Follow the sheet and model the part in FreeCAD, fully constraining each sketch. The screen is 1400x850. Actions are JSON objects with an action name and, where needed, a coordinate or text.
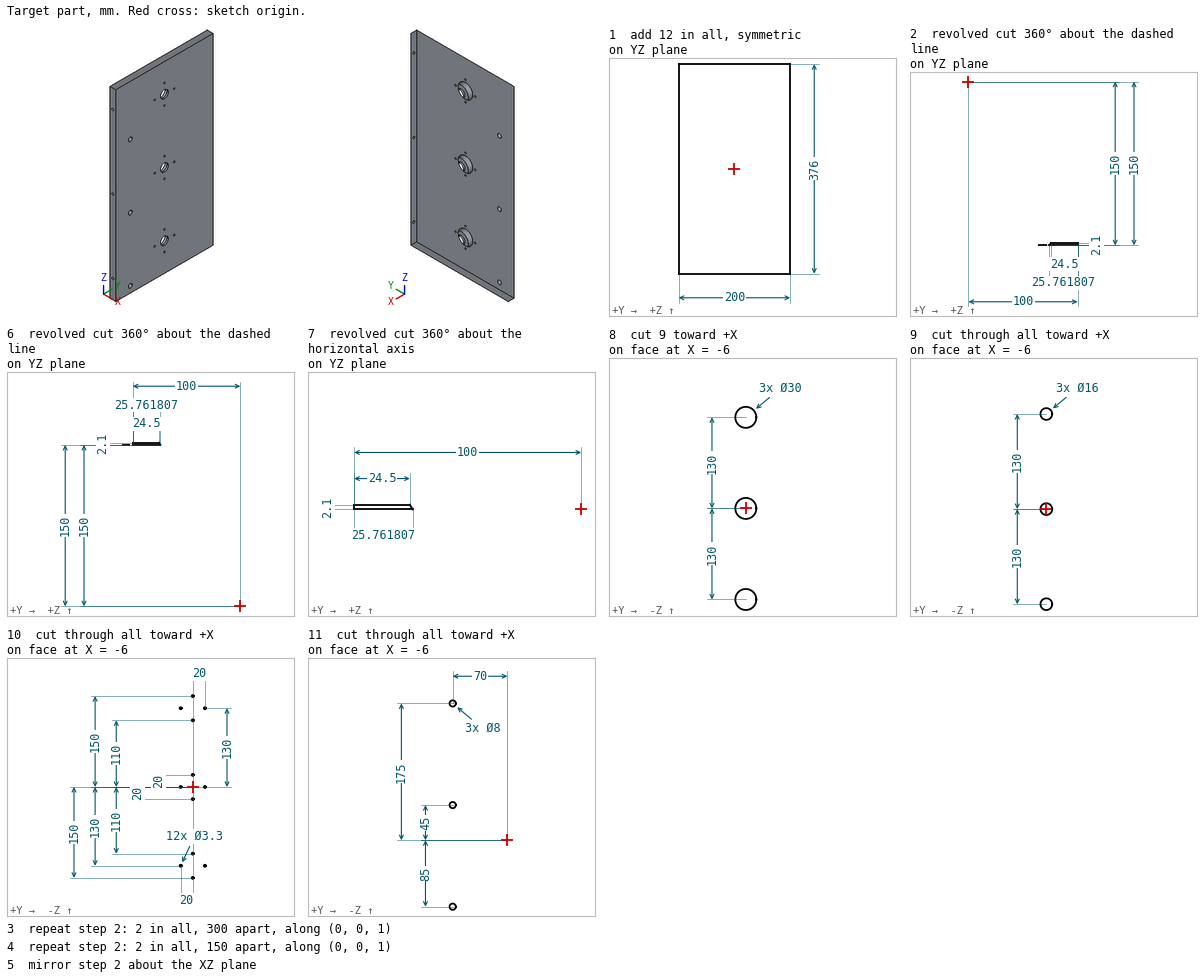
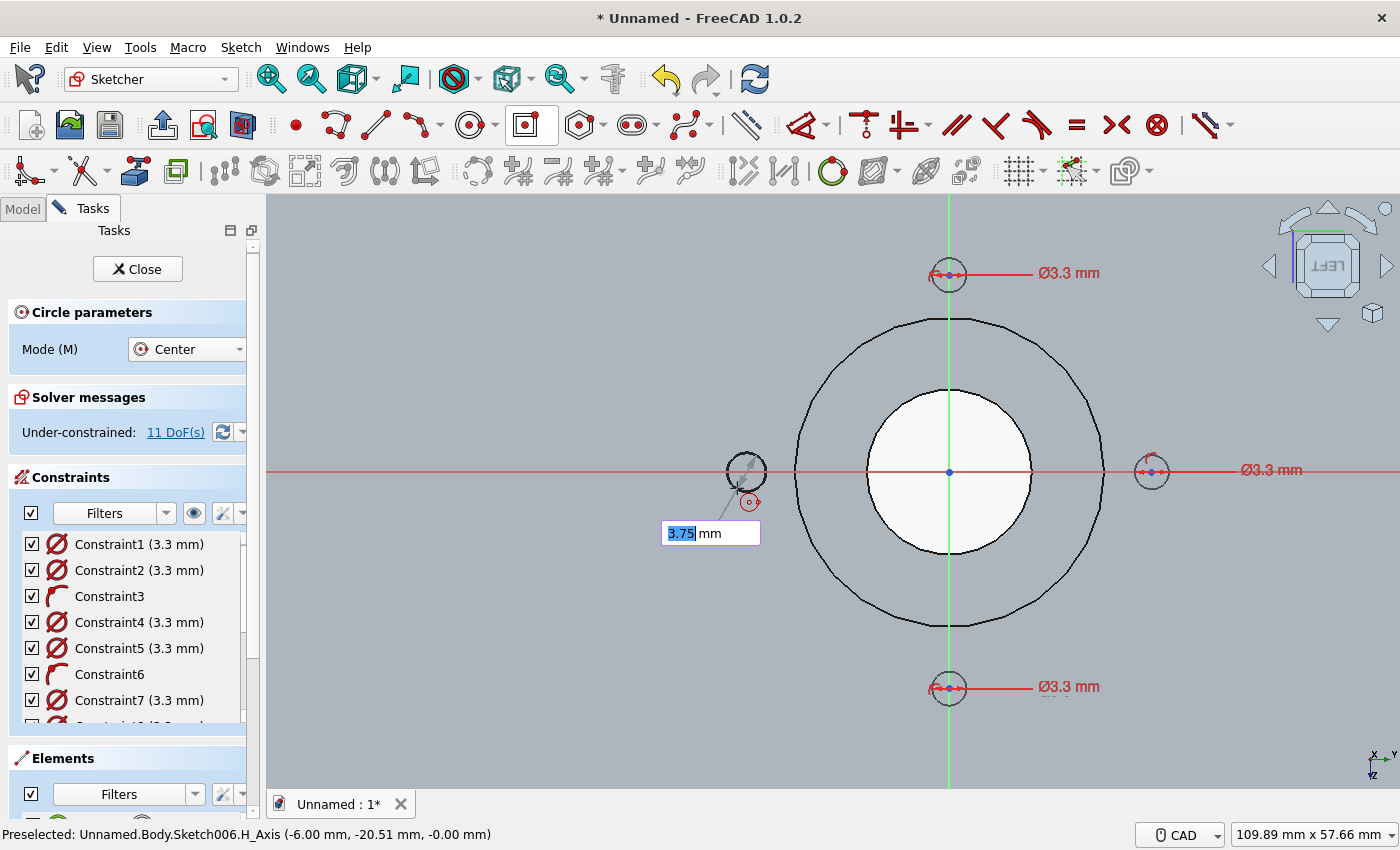
{"action": "type", "text": "3.3"}
{"action": "key", "text": "Return"}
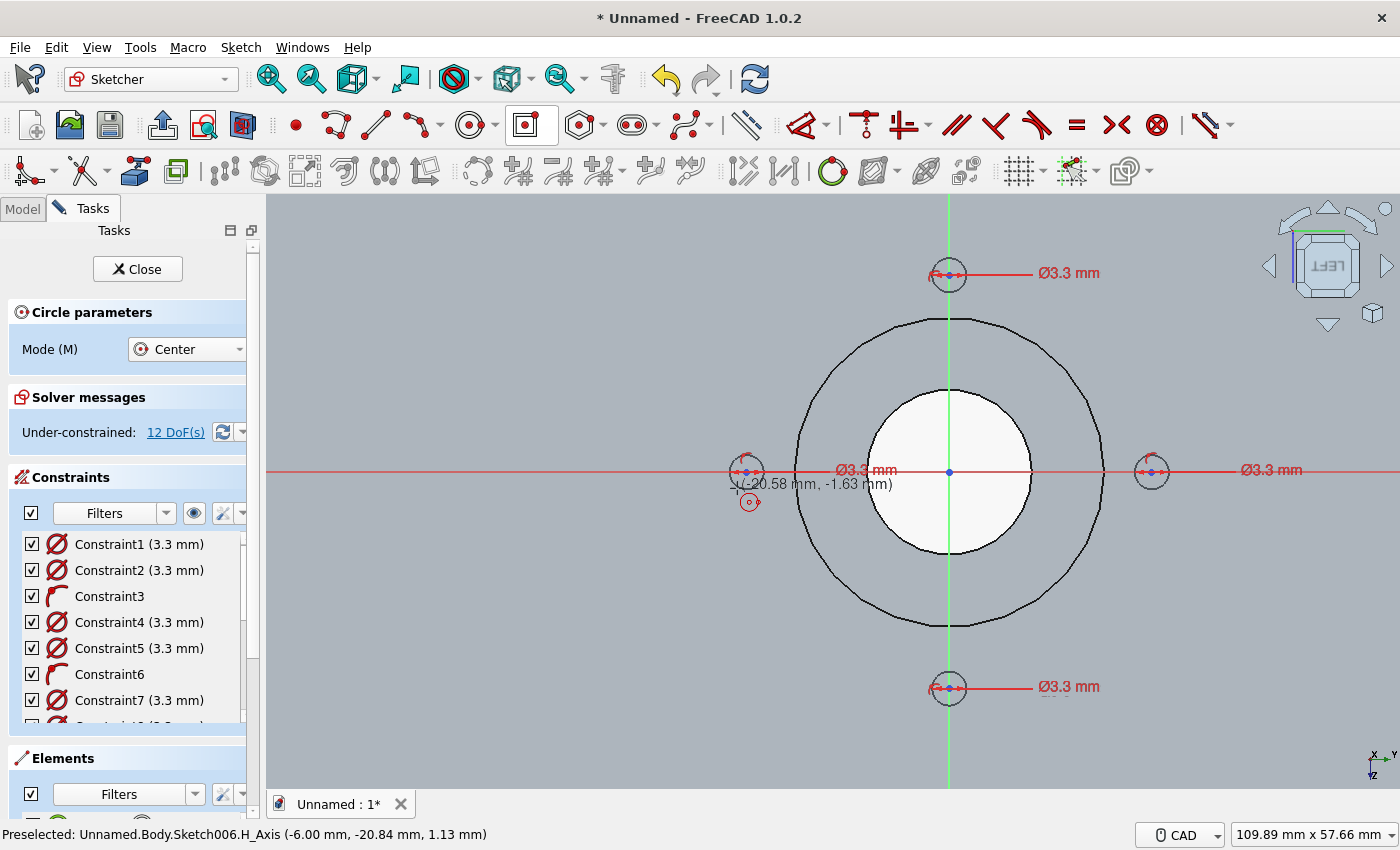
{"action": "scroll", "coordinate": [741, 494], "scroll_direction": "down", "scroll_amount": 11}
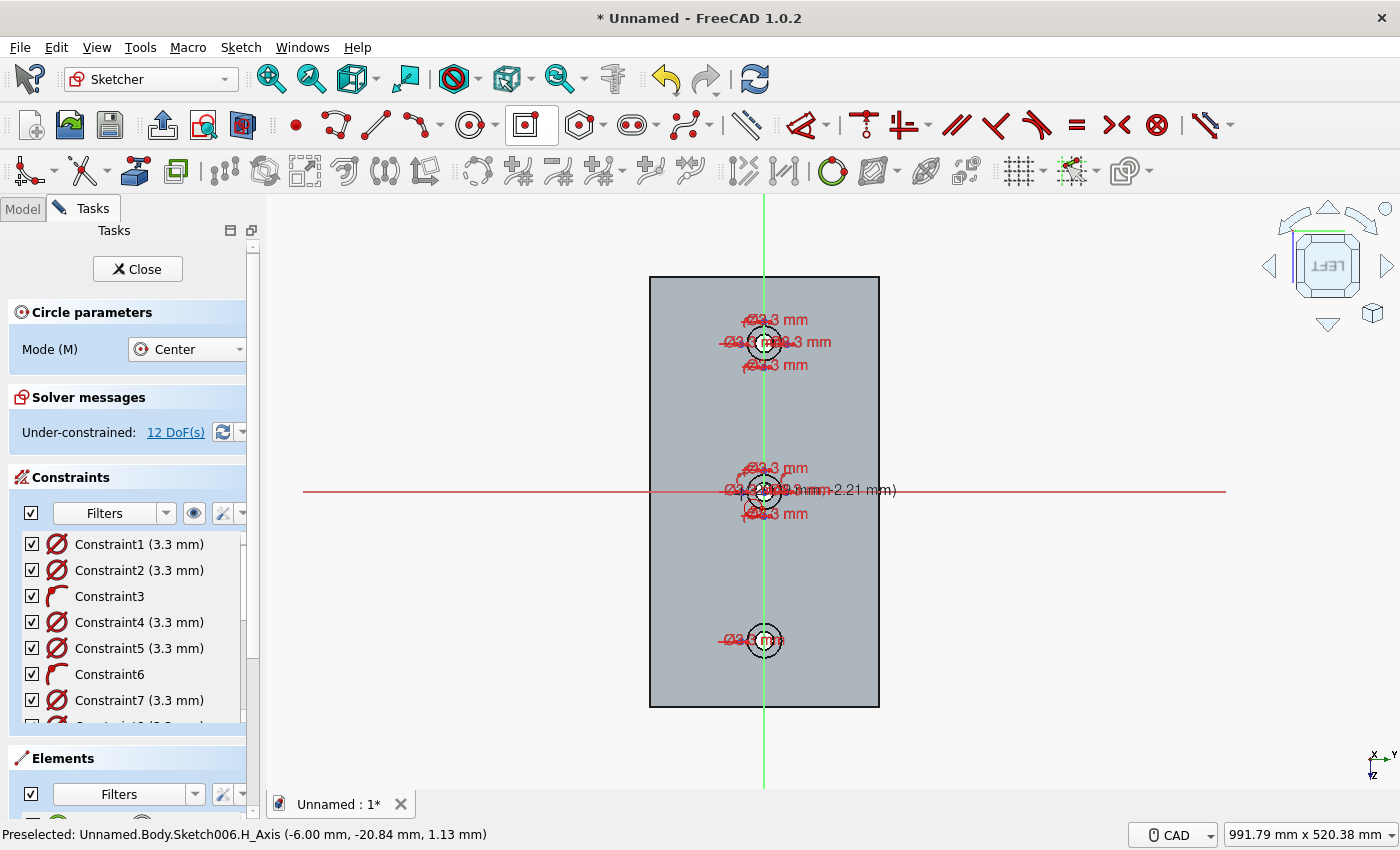
{"action": "scroll", "coordinate": [764, 618], "scroll_direction": "up", "scroll_amount": 13}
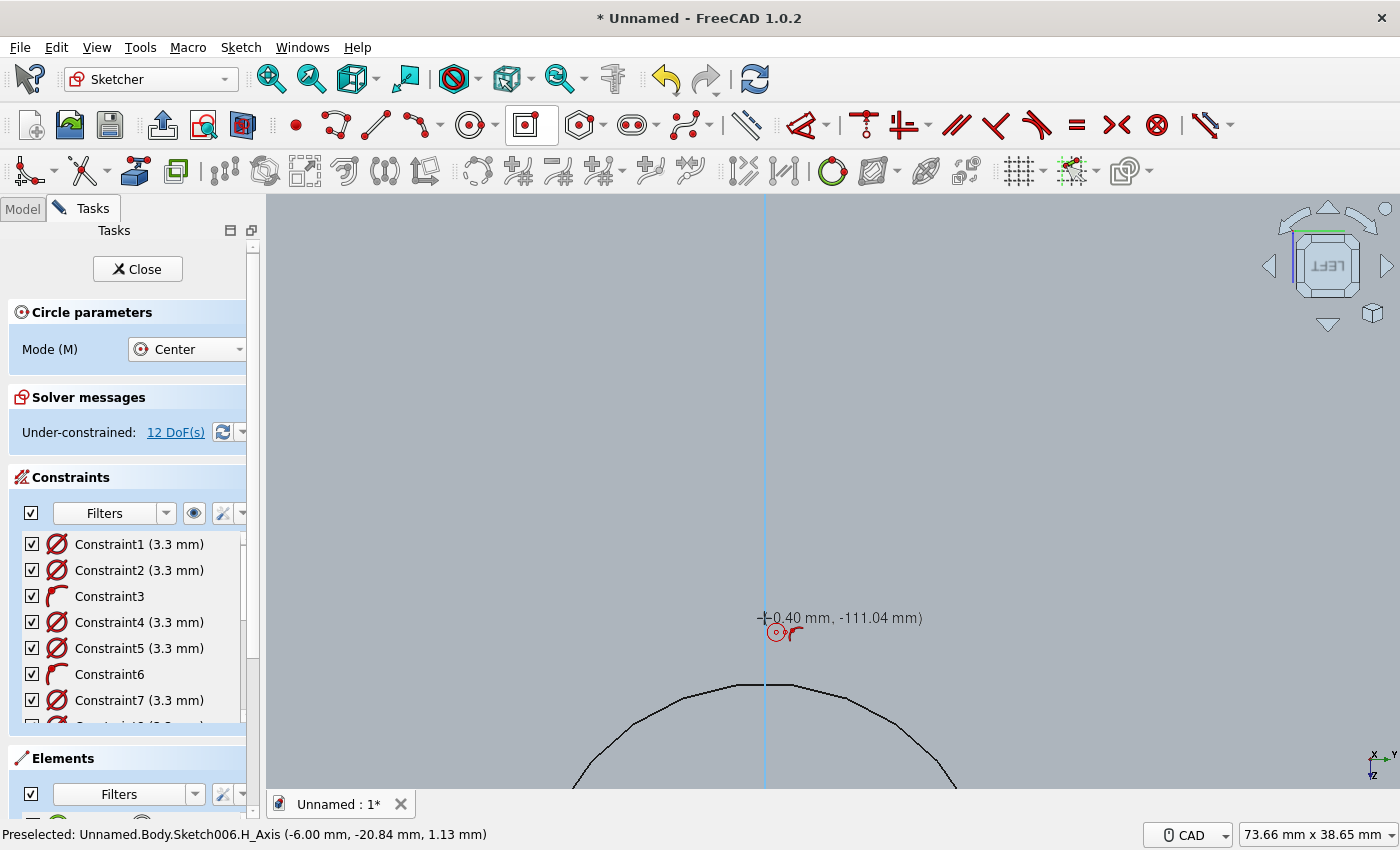
{"action": "scroll", "coordinate": [764, 618], "scroll_direction": "down", "scroll_amount": 13}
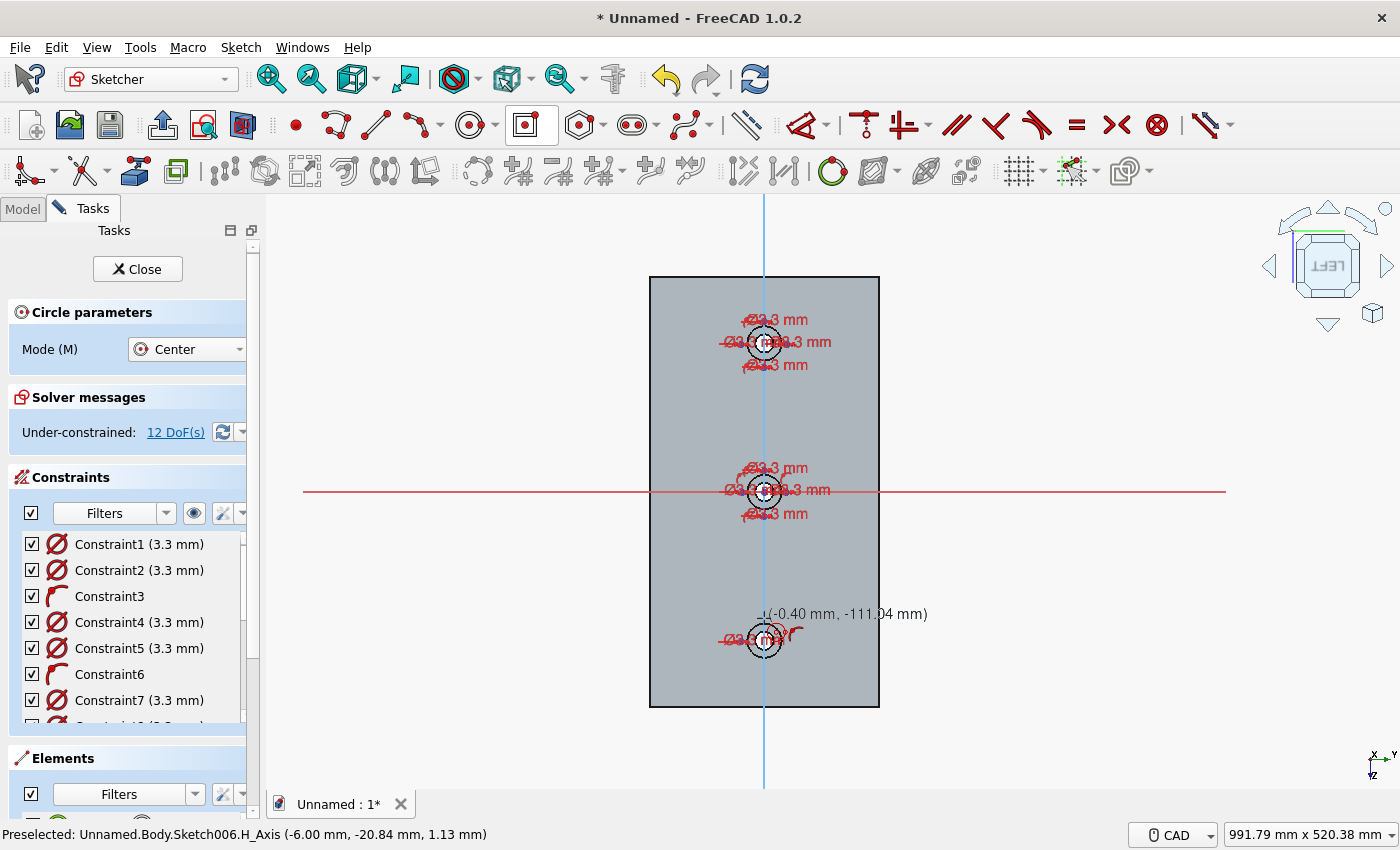
{"action": "left_click", "coordinate": [764, 618]}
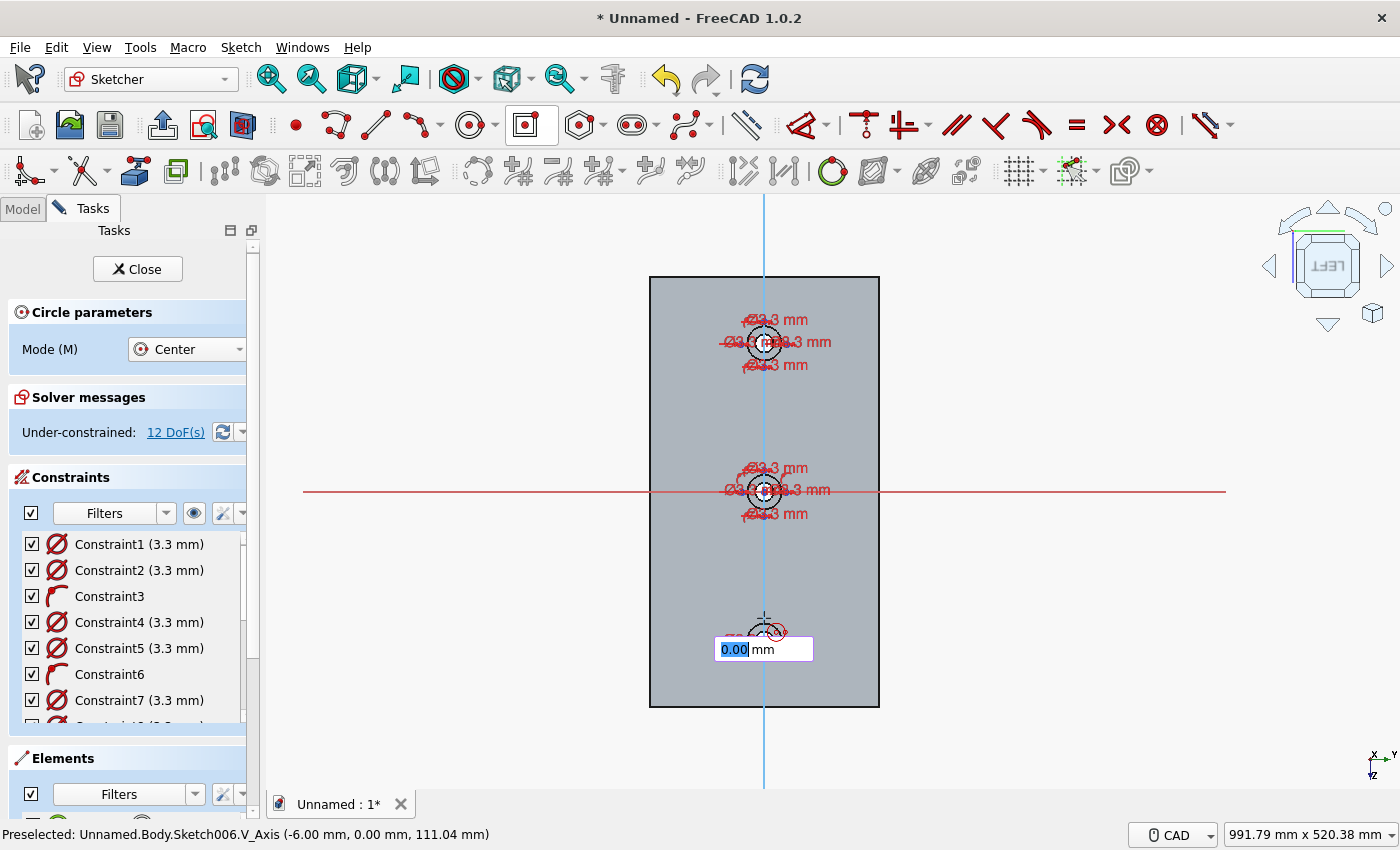
{"action": "scroll", "coordinate": [766, 617], "scroll_direction": "up", "scroll_amount": 11}
{"action": "mouse_move", "coordinate": [765, 613]}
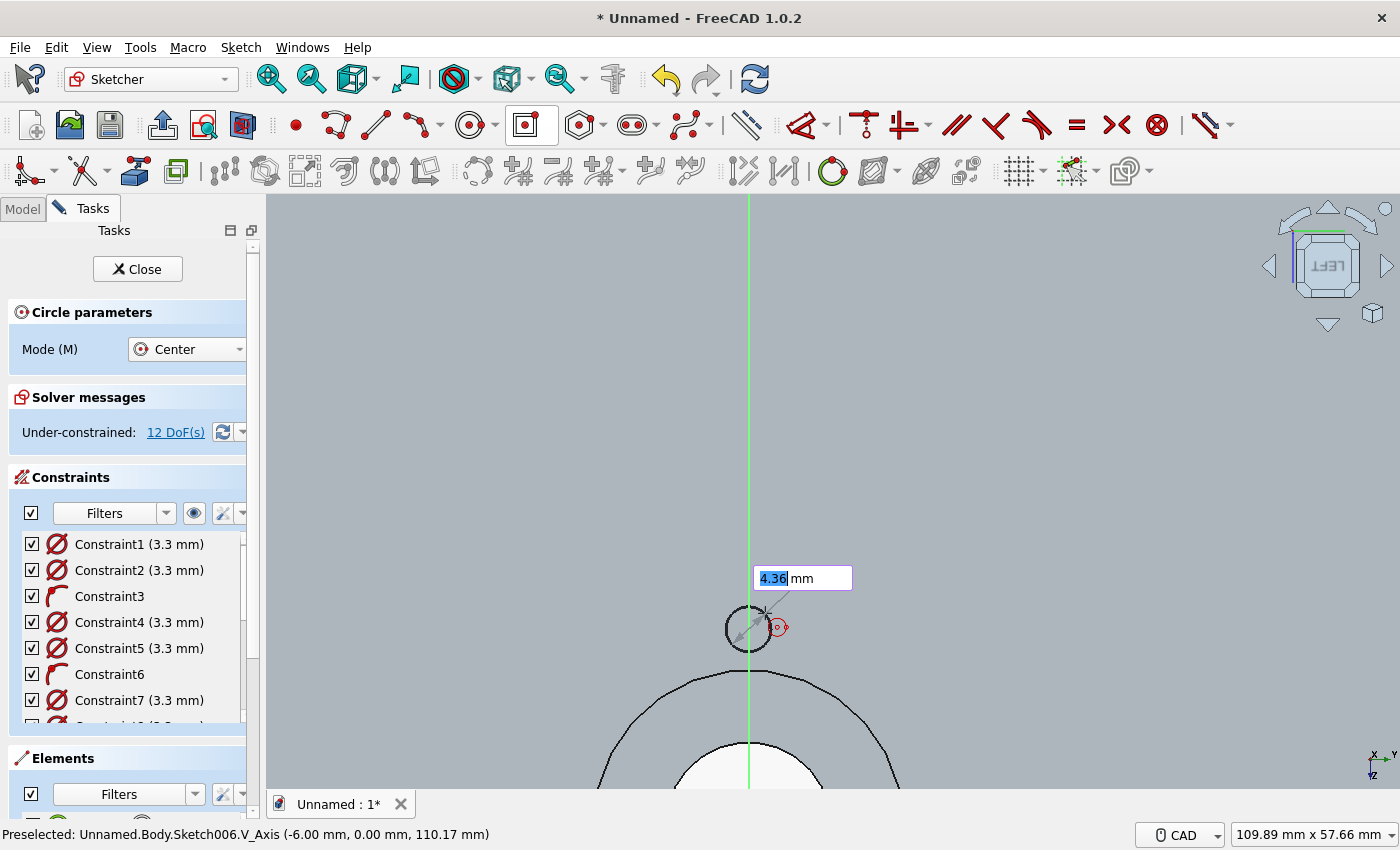
{"action": "type", "text": "3.3"}
{"action": "key", "text": "Return"}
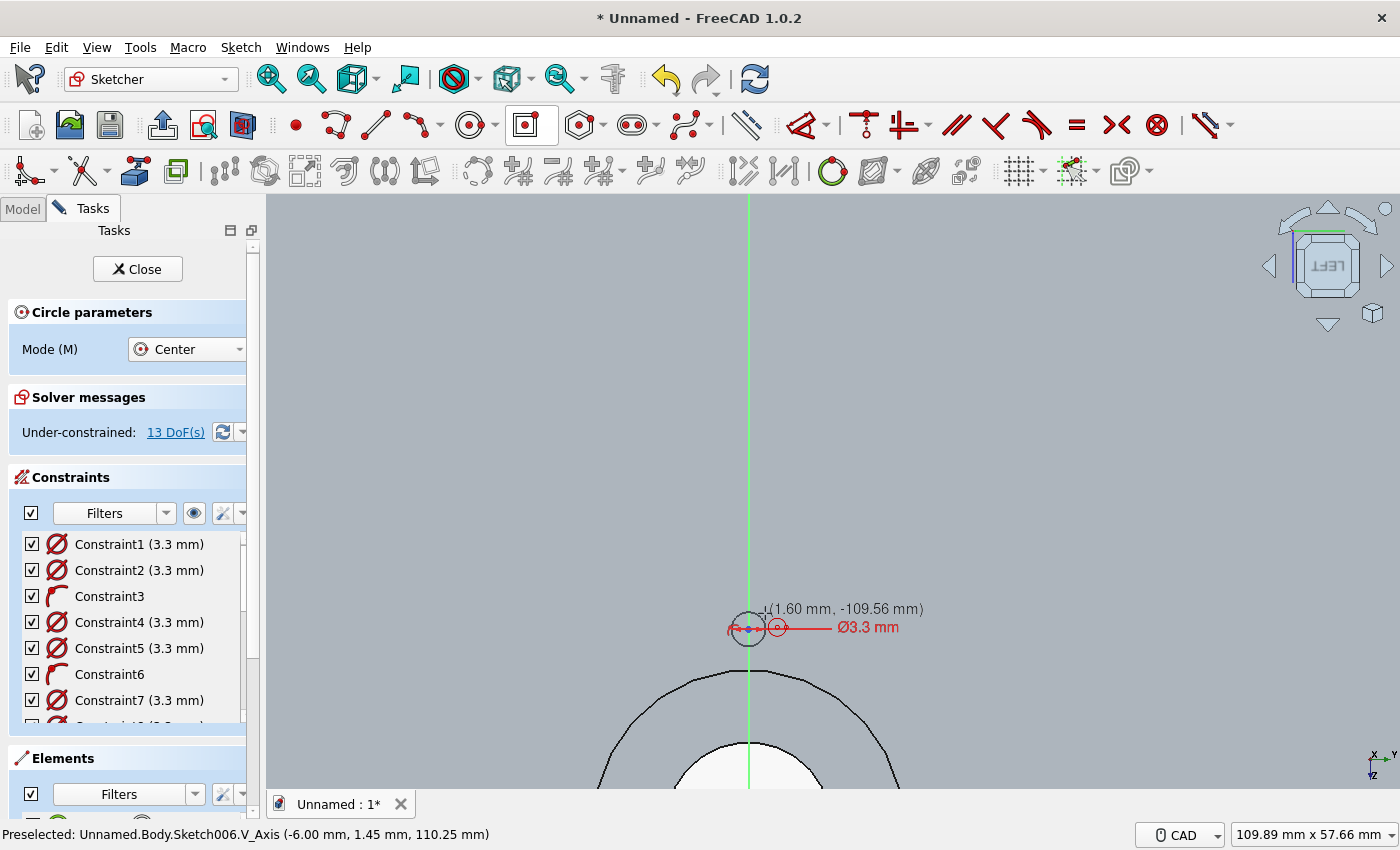
{"action": "scroll", "coordinate": [766, 617], "scroll_direction": "down", "scroll_amount": 11}